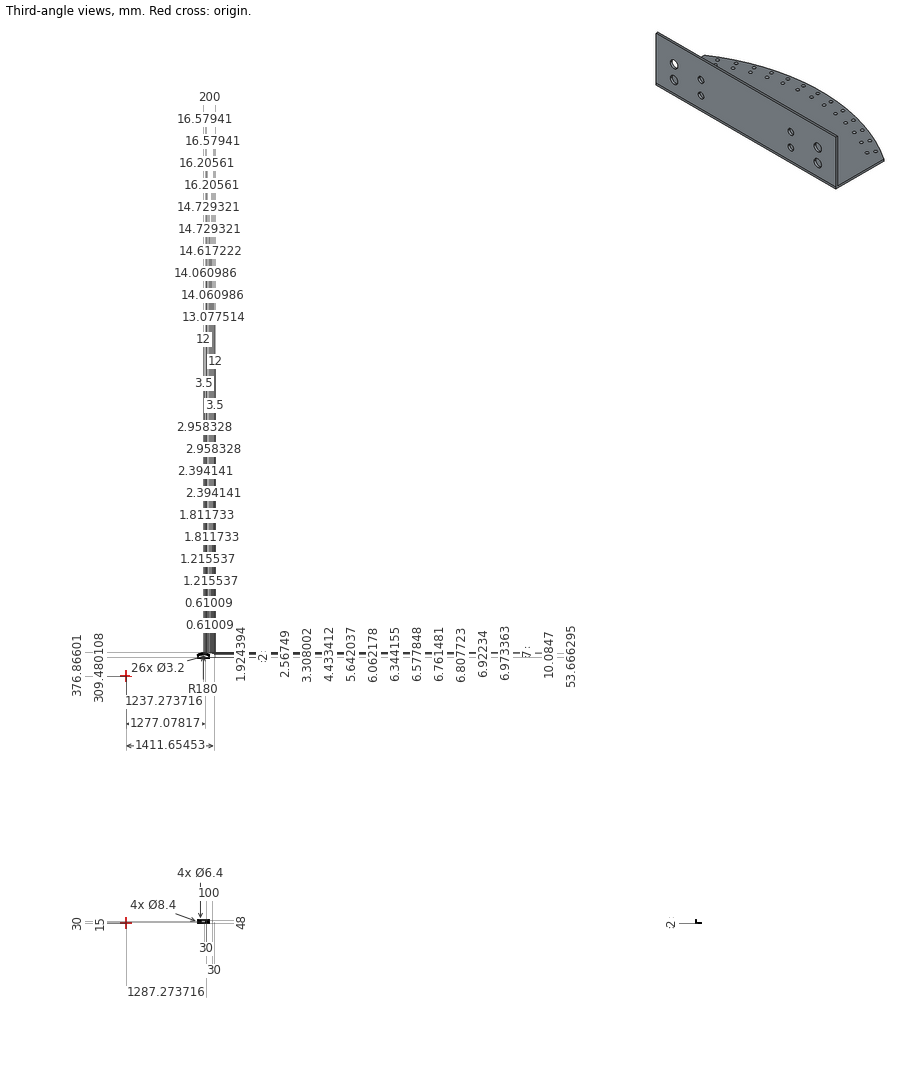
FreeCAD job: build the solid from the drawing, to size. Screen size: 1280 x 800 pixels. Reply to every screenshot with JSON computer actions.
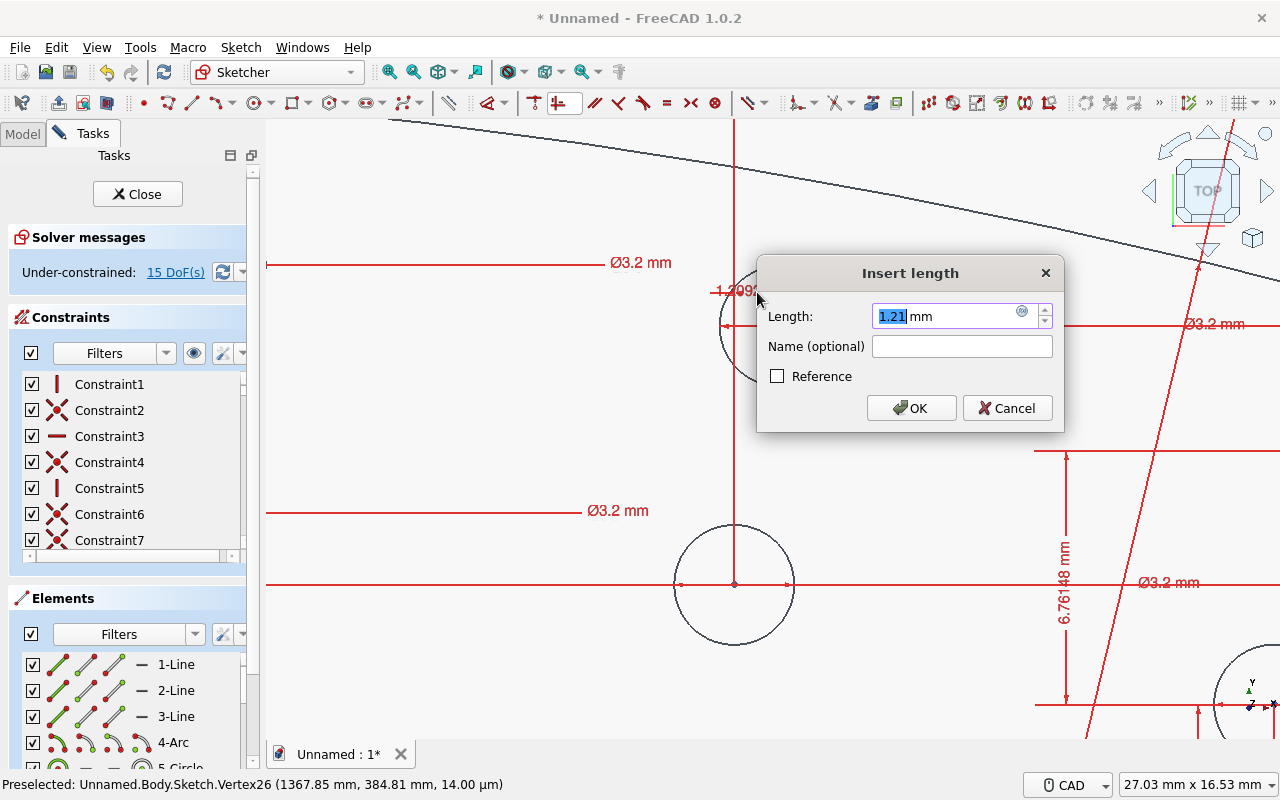
{"action": "type", "text": "1.215537"}
{"action": "key", "text": "Return"}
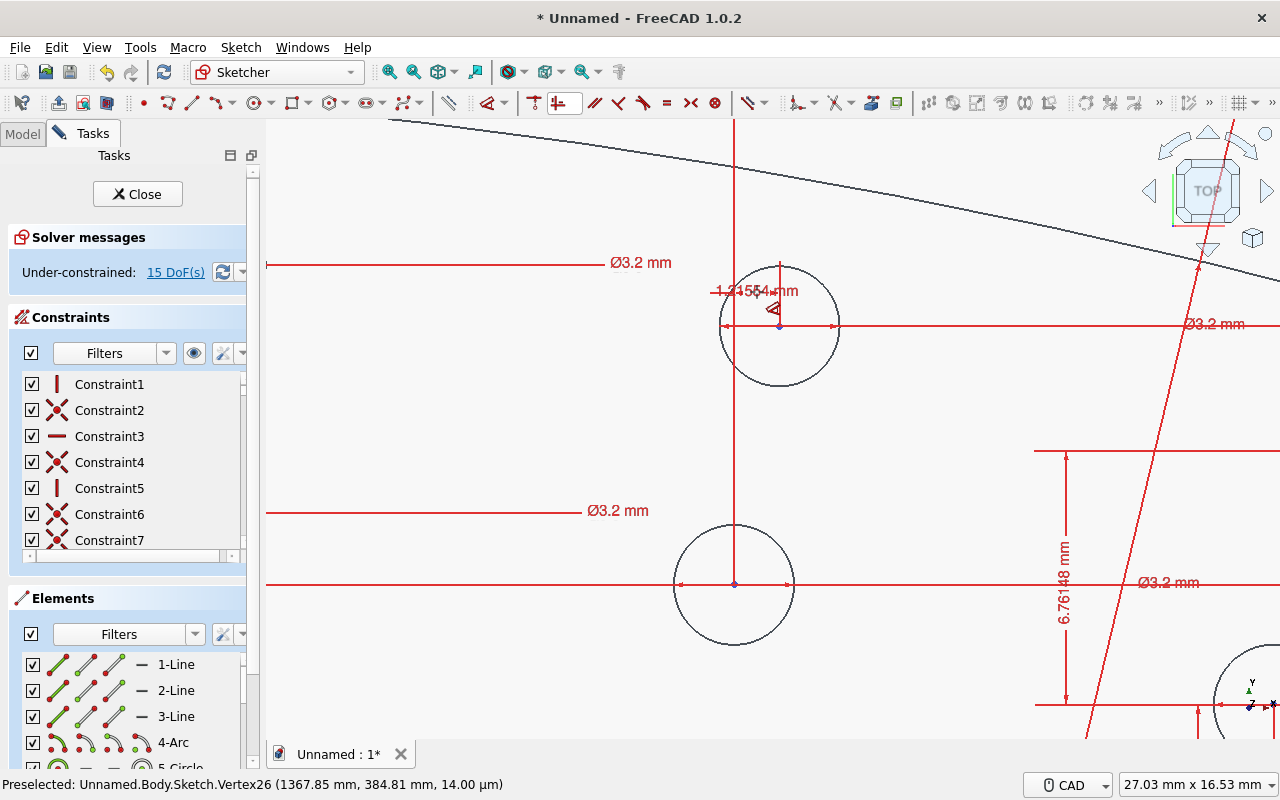
{"action": "scroll", "coordinate": [791, 331], "scroll_direction": "down", "scroll_amount": 13}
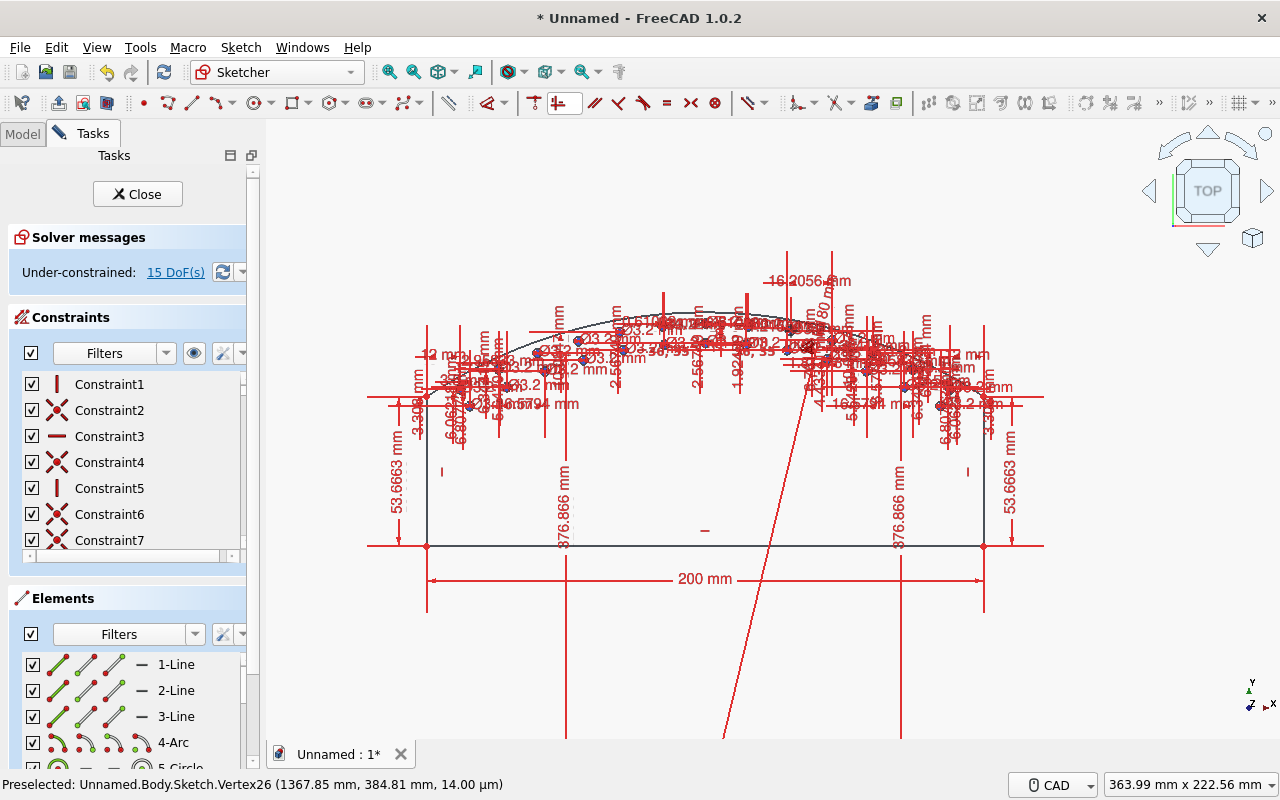
{"action": "scroll", "coordinate": [746, 345], "scroll_direction": "up", "scroll_amount": 4}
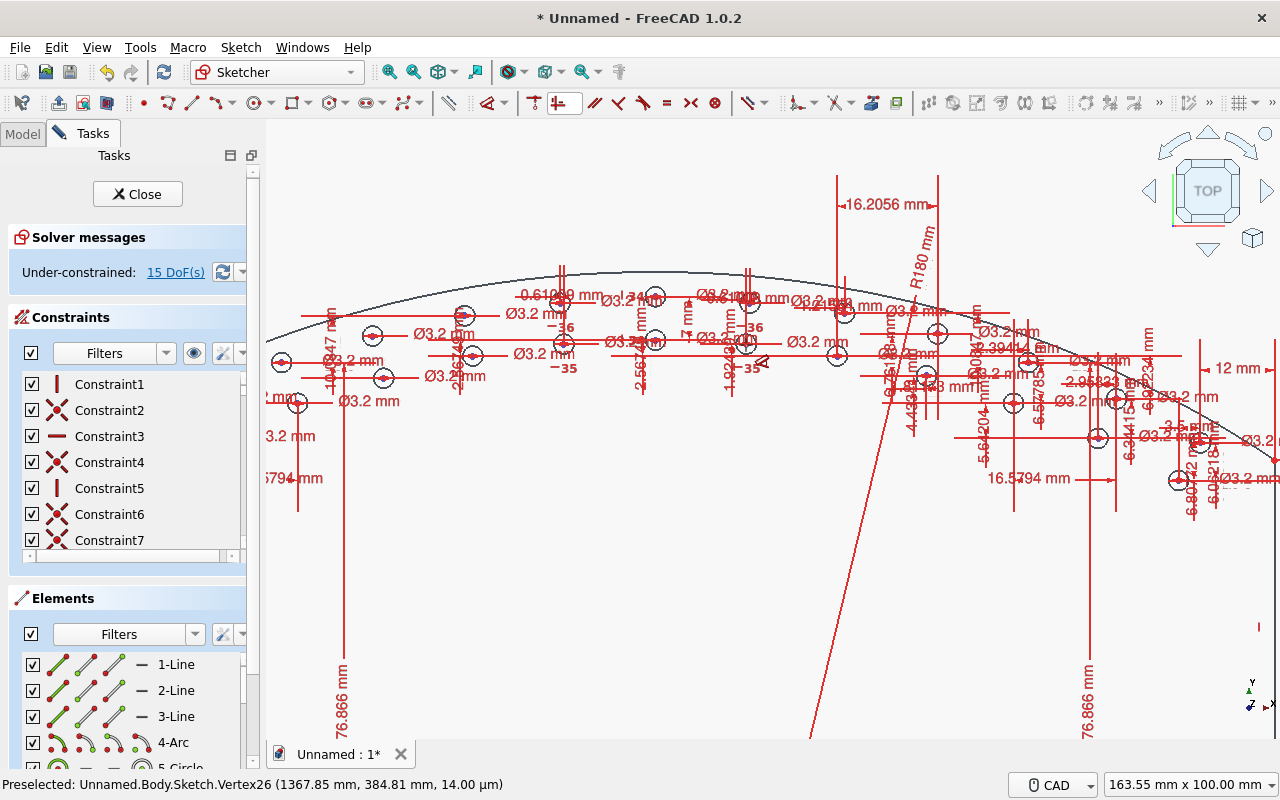
{"action": "left_click", "coordinate": [746, 344]}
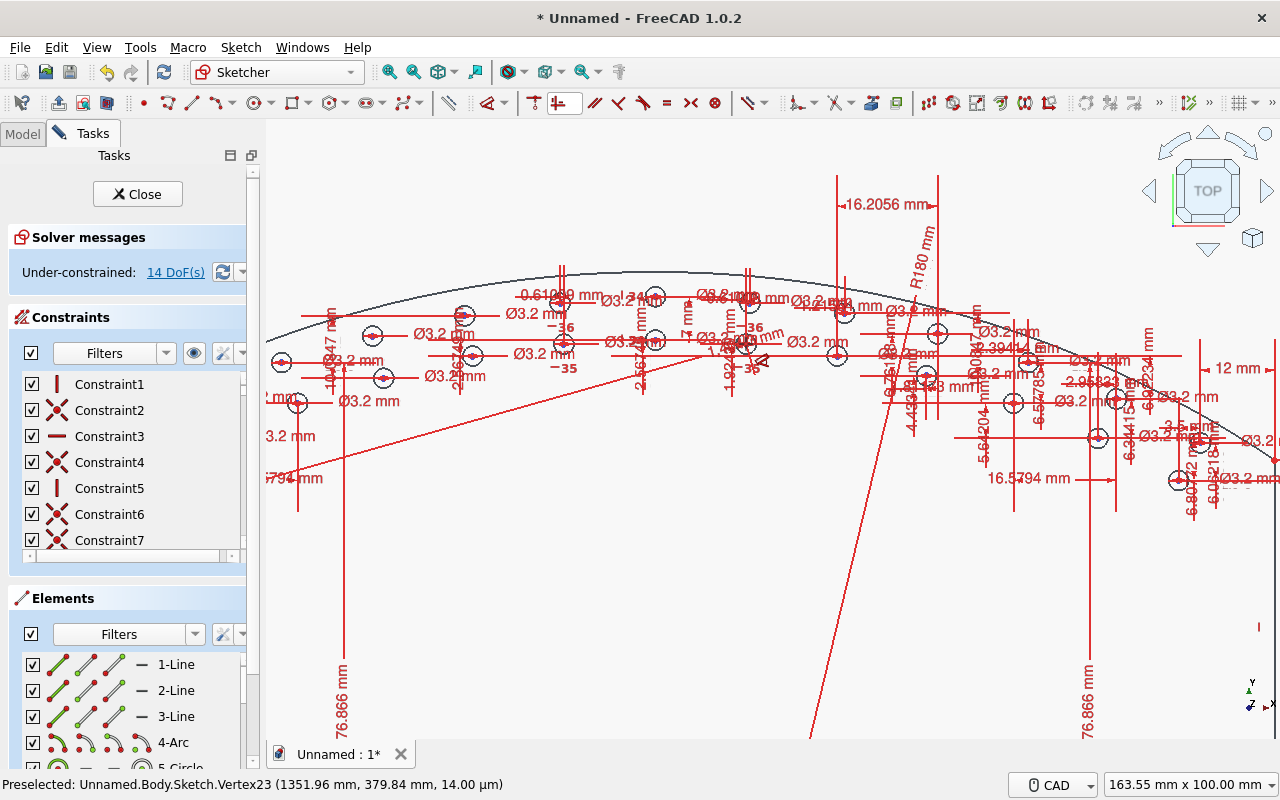
{"action": "left_click", "coordinate": [750, 303]}
{"action": "left_click", "coordinate": [808, 333]}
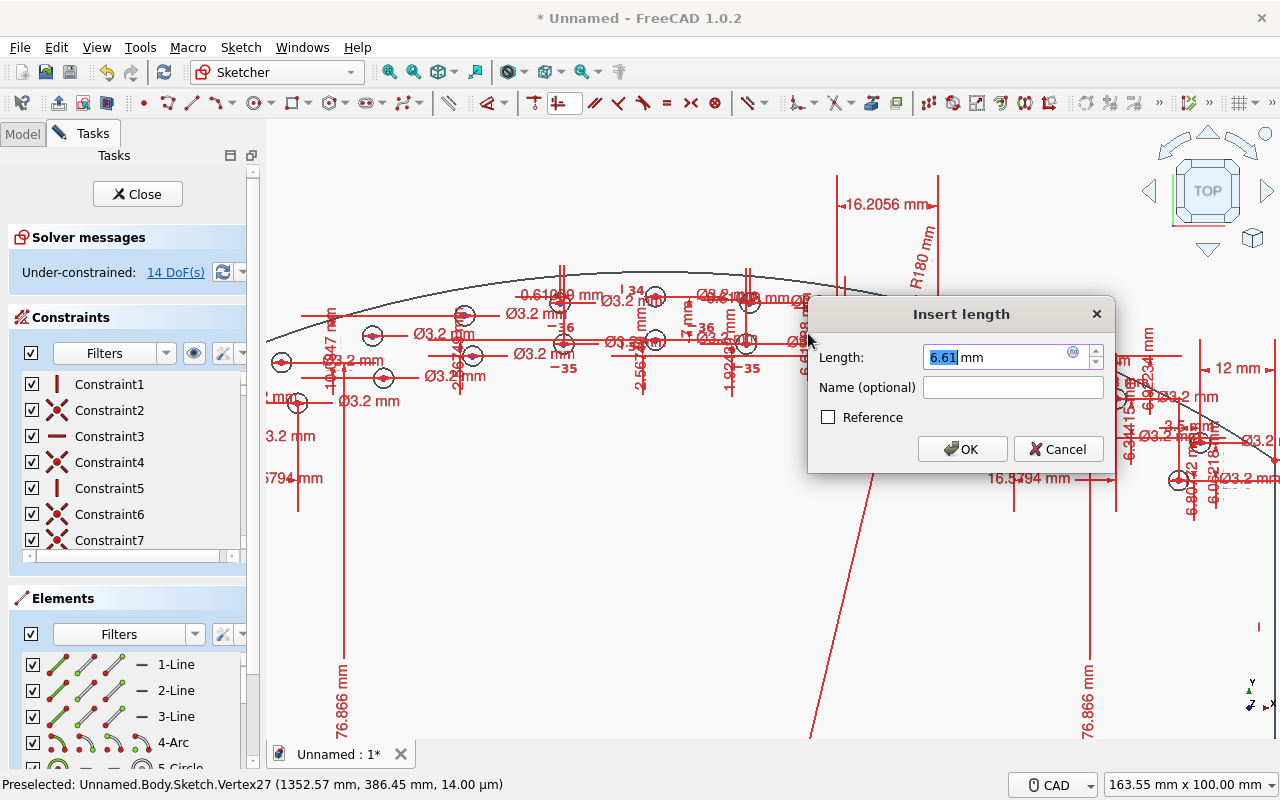
{"action": "type", "text": "6.973363"}
{"action": "key", "text": "Return"}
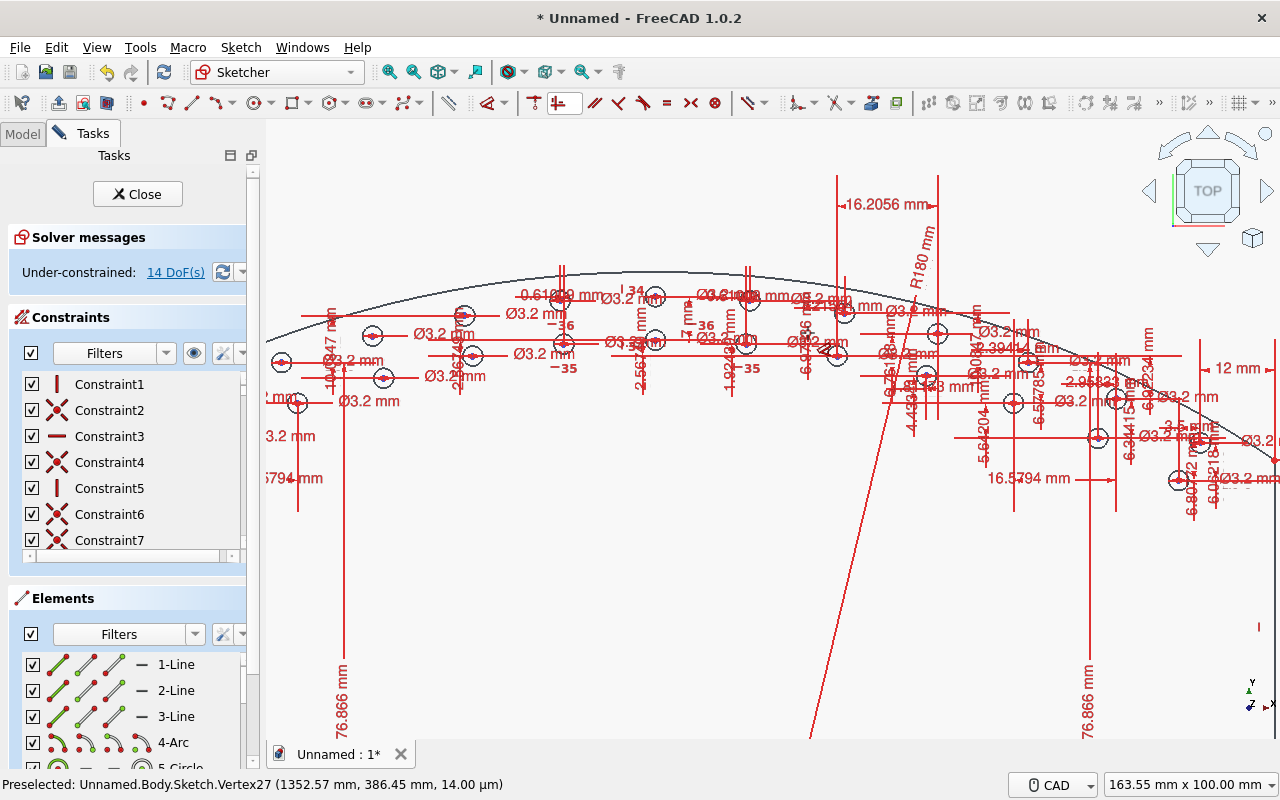
{"action": "scroll", "coordinate": [298, 403], "scroll_direction": "up", "scroll_amount": 2}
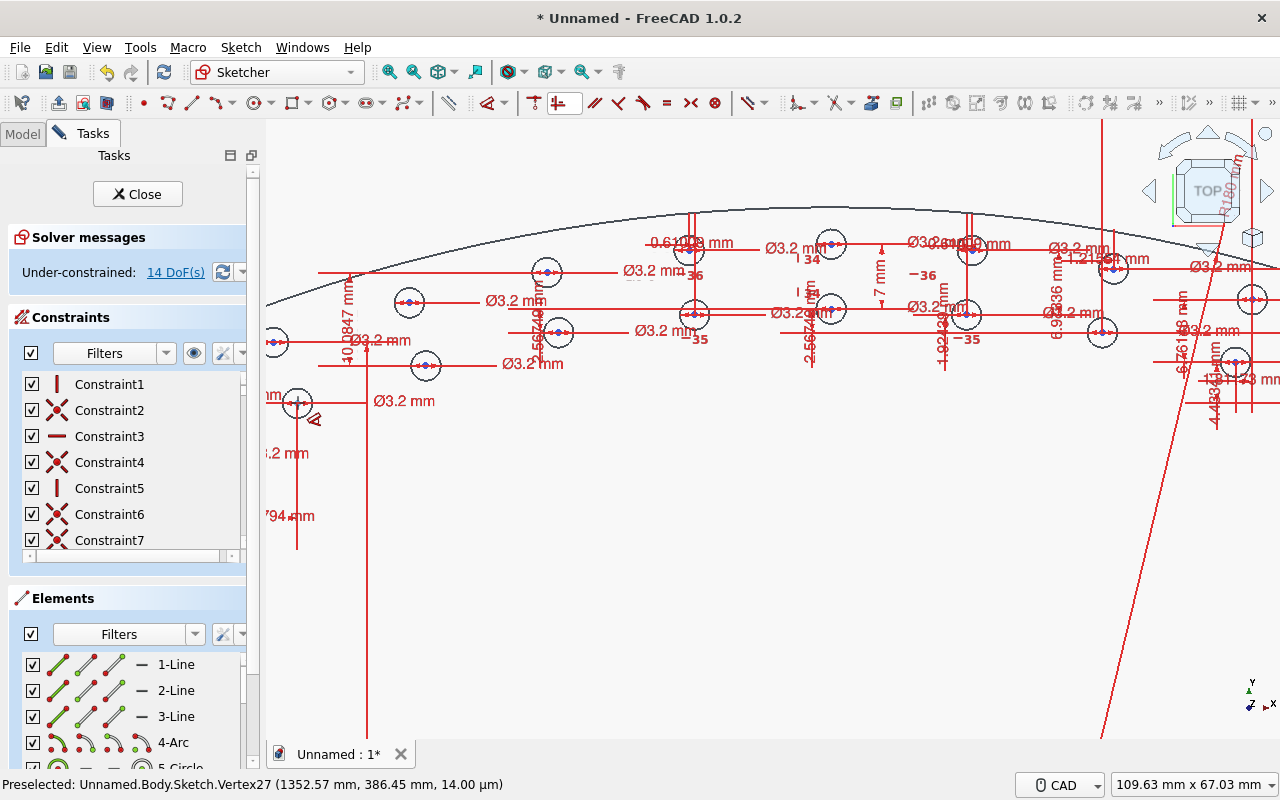
{"action": "left_click", "coordinate": [297, 403]}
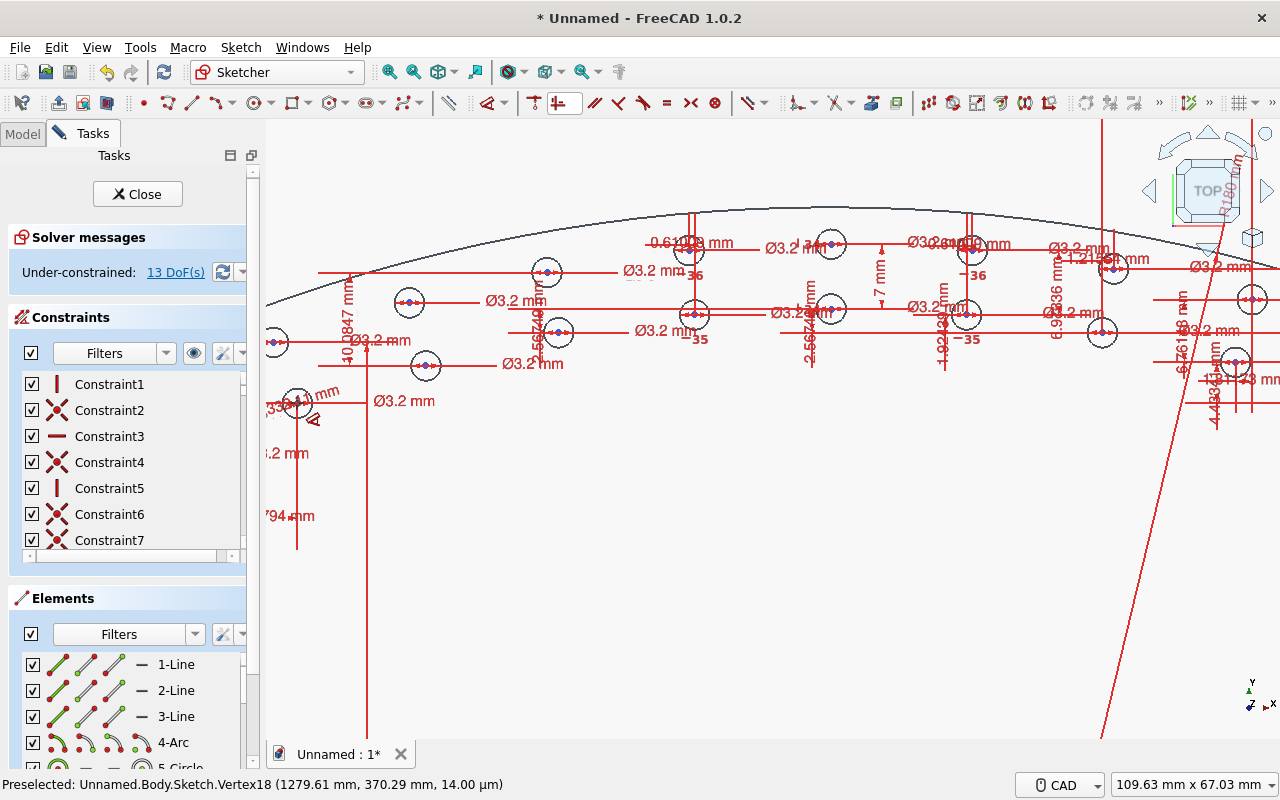
{"action": "left_click", "coordinate": [426, 366]}
{"action": "left_click", "coordinate": [460, 385]}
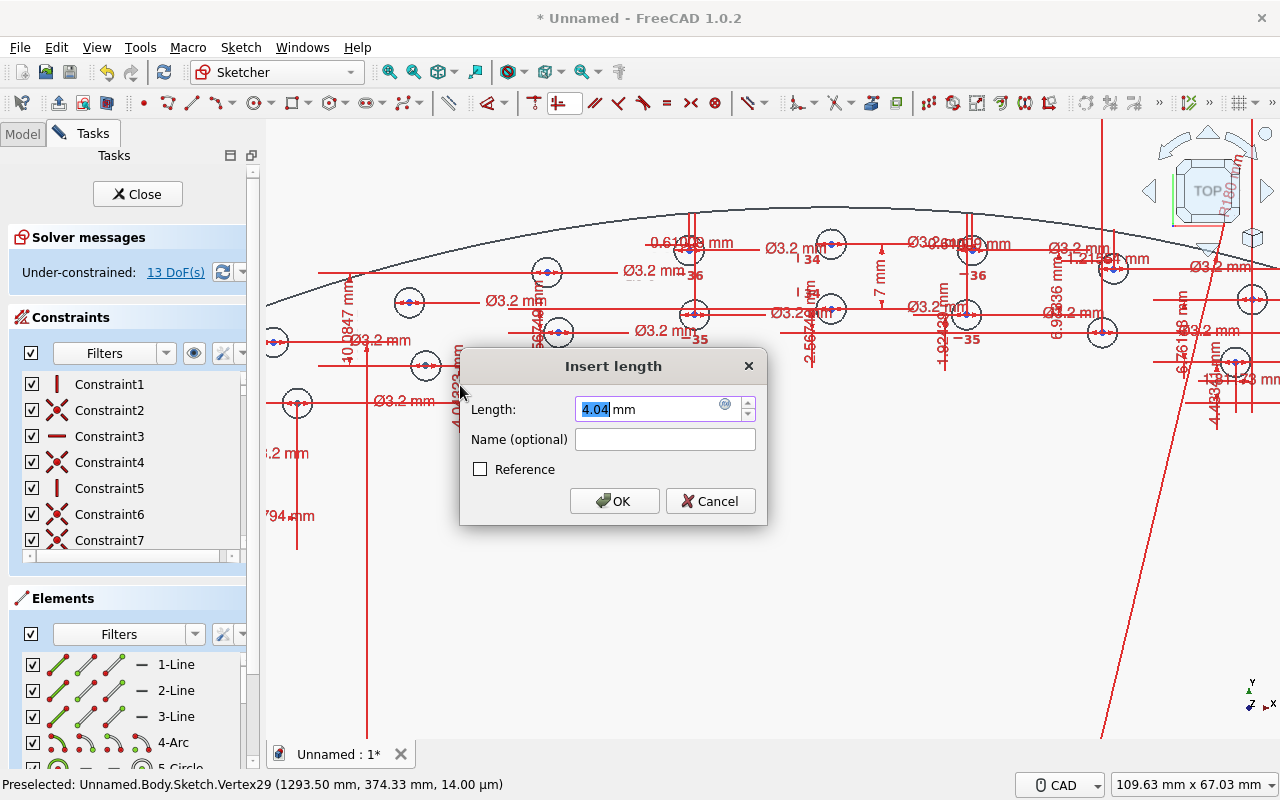
{"action": "type", "text": "4.433412"}
{"action": "key", "text": "Return"}